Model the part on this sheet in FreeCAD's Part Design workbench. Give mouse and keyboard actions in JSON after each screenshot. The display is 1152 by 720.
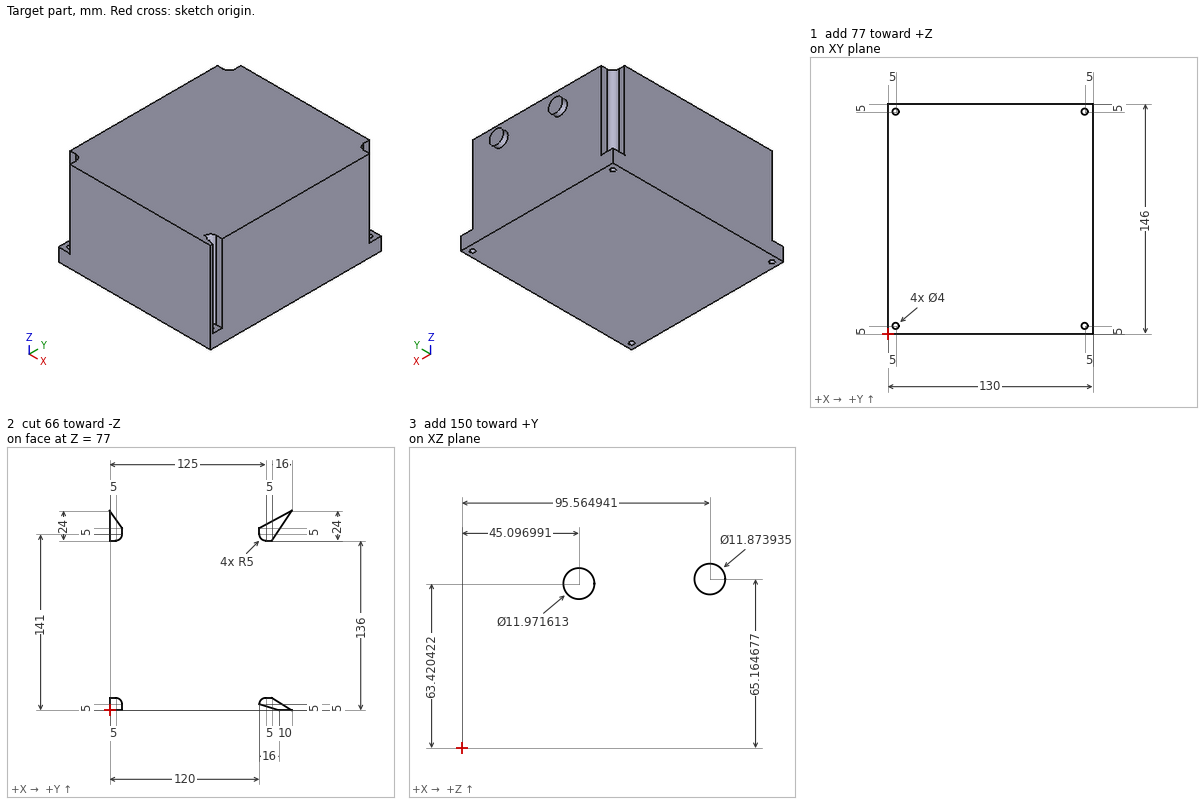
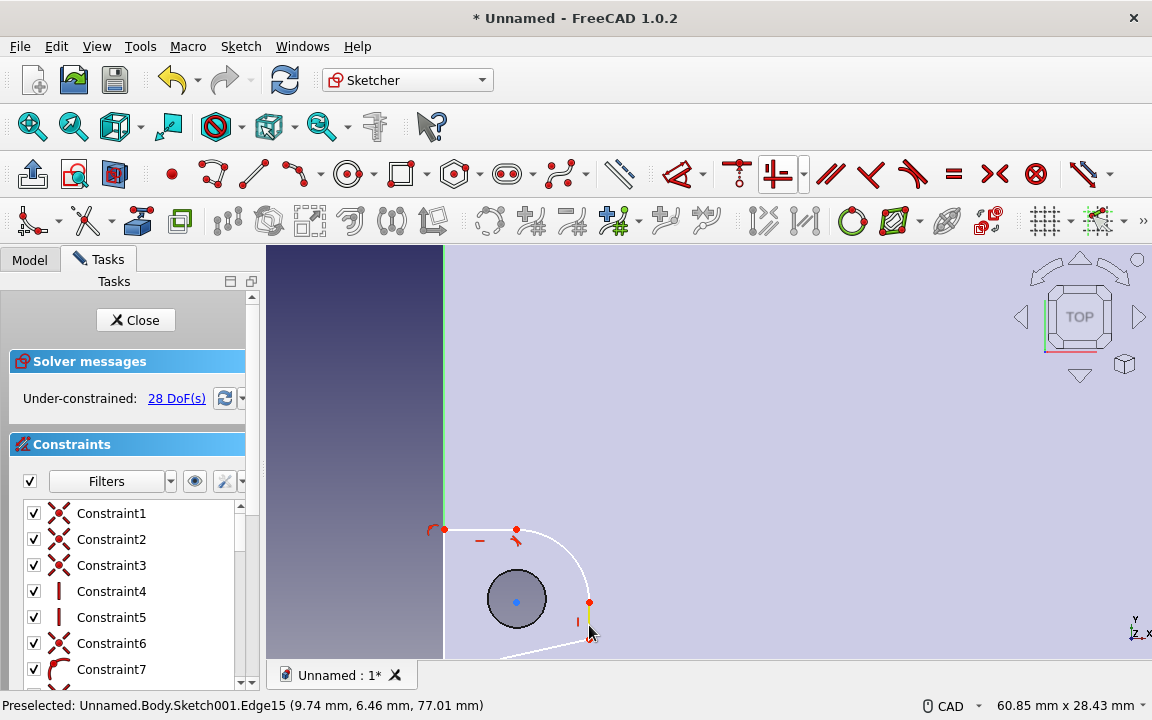
{"action": "left_click", "coordinate": [589, 625]}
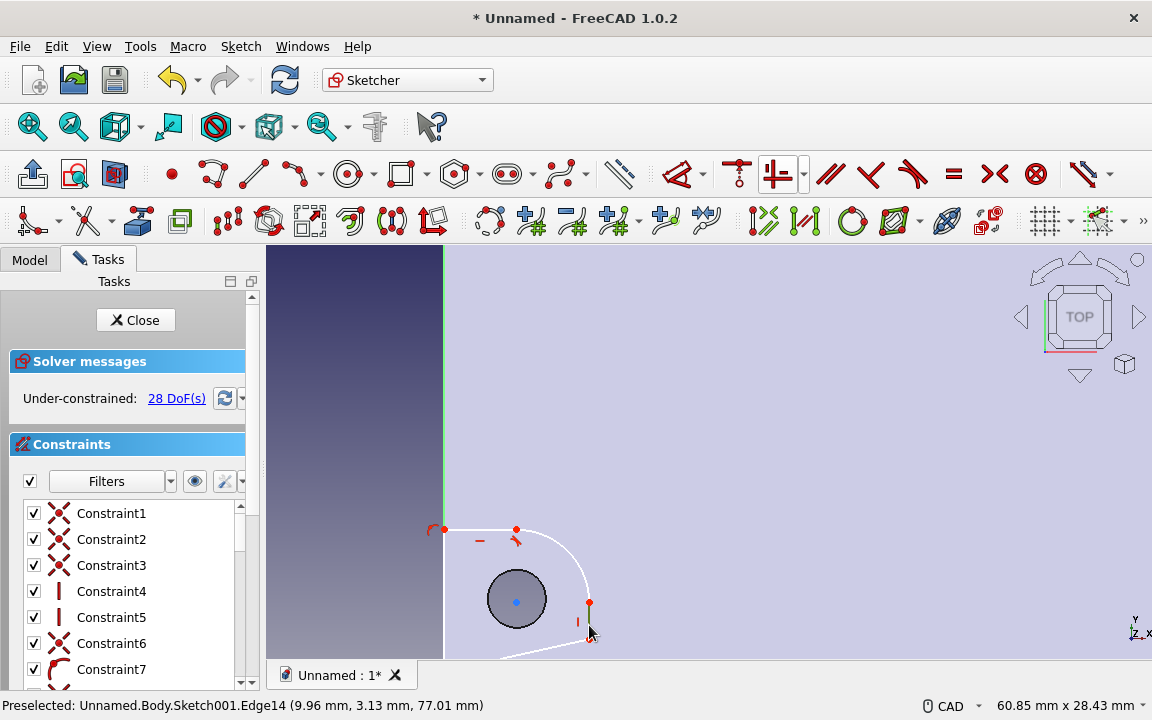
{"action": "left_click", "coordinate": [581, 570]}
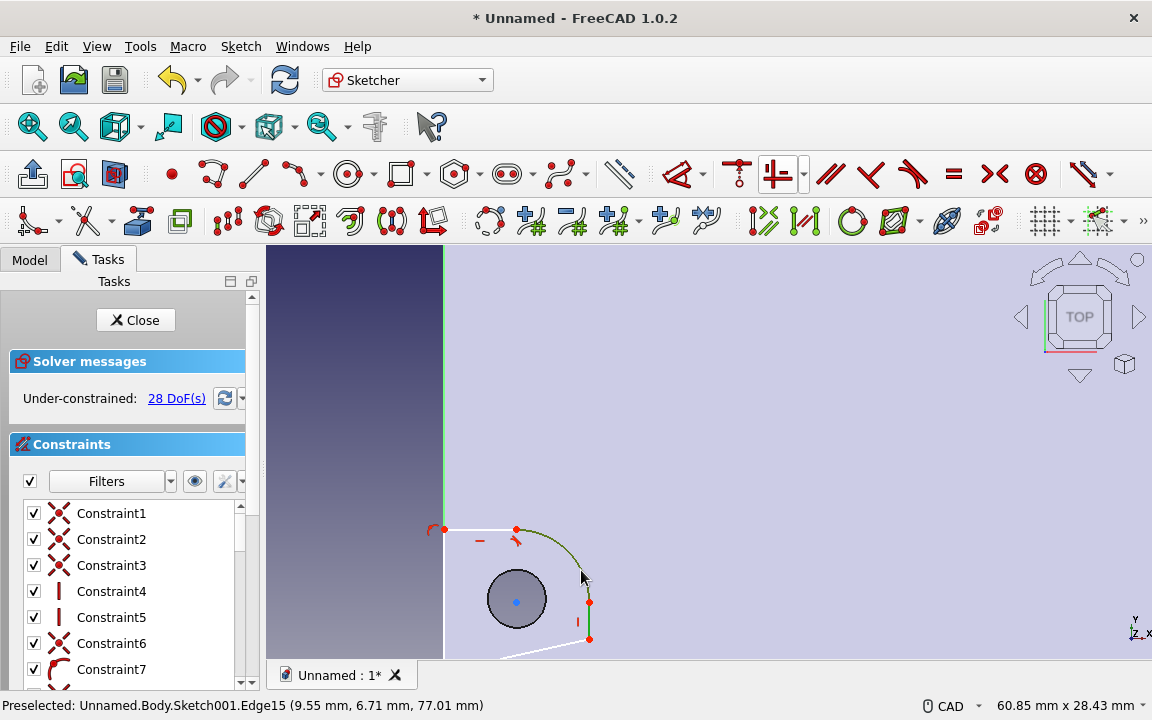
{"action": "left_click", "coordinate": [913, 174]}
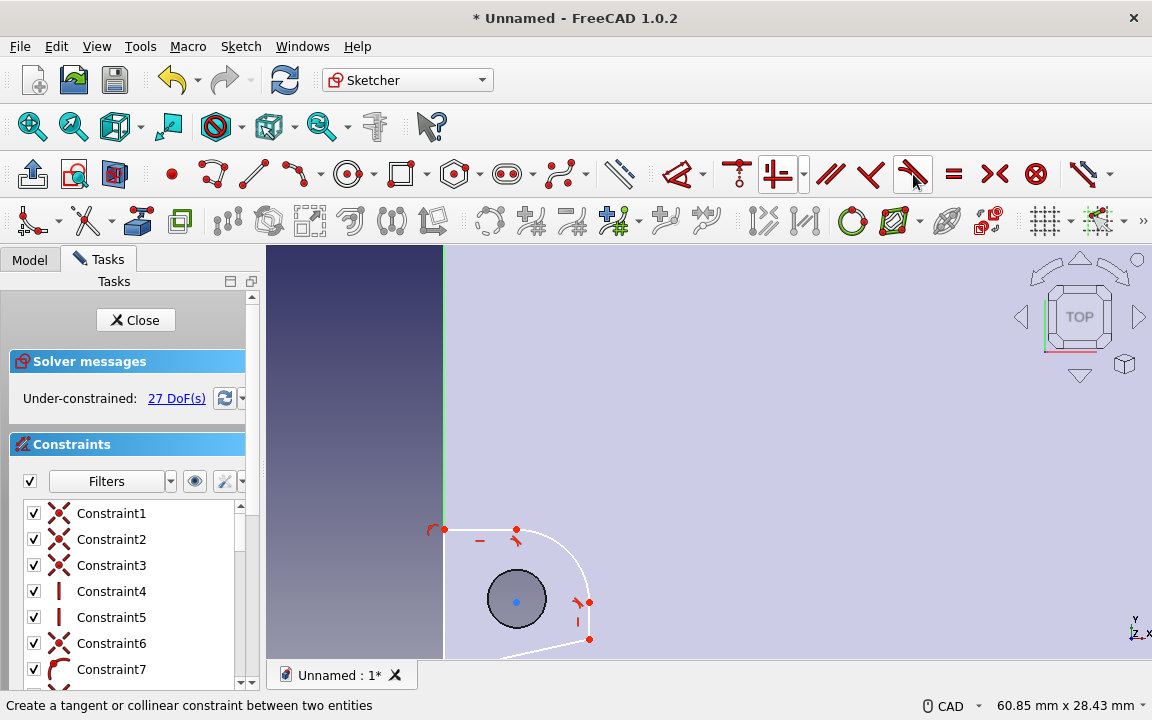
{"action": "scroll", "coordinate": [533, 570], "scroll_direction": "down", "scroll_amount": 11}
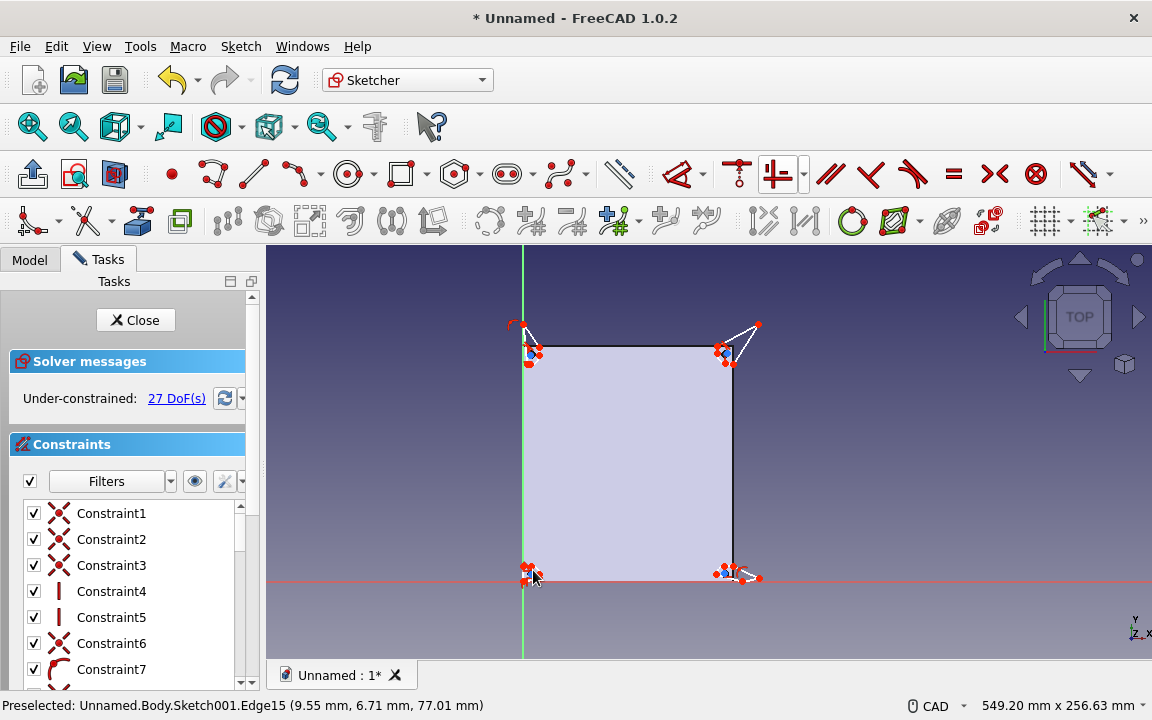
{"action": "scroll", "coordinate": [731, 566], "scroll_direction": "up", "scroll_amount": 9}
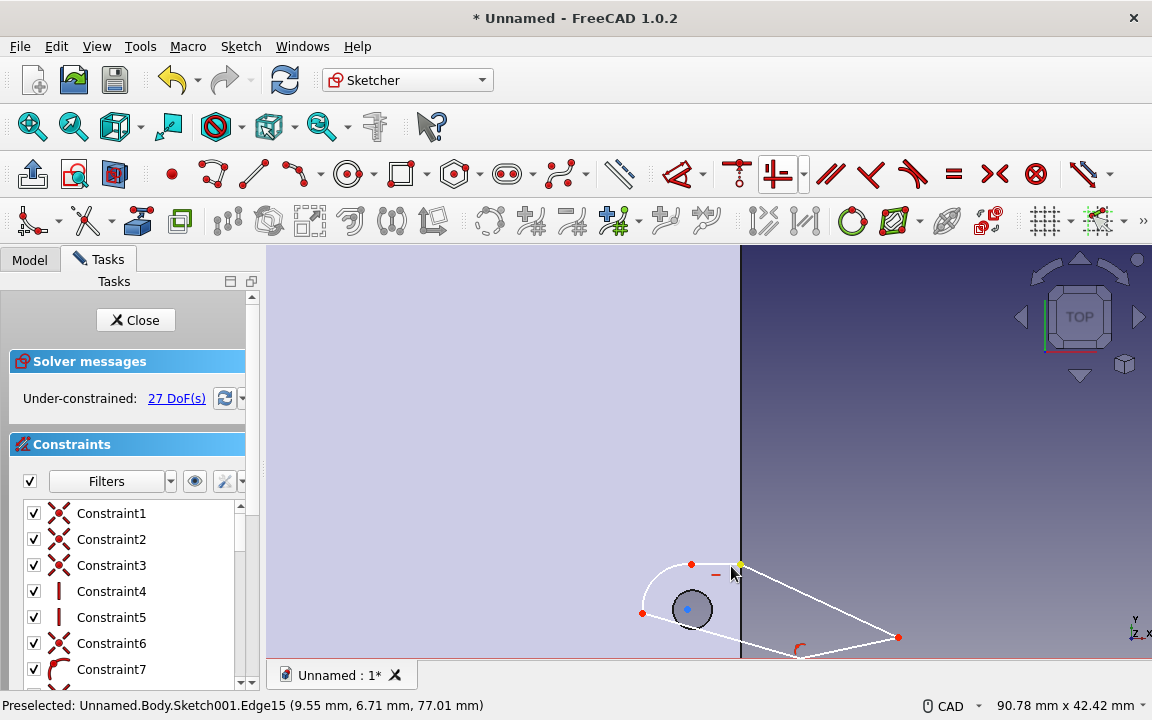
{"action": "left_click", "coordinate": [726, 564]}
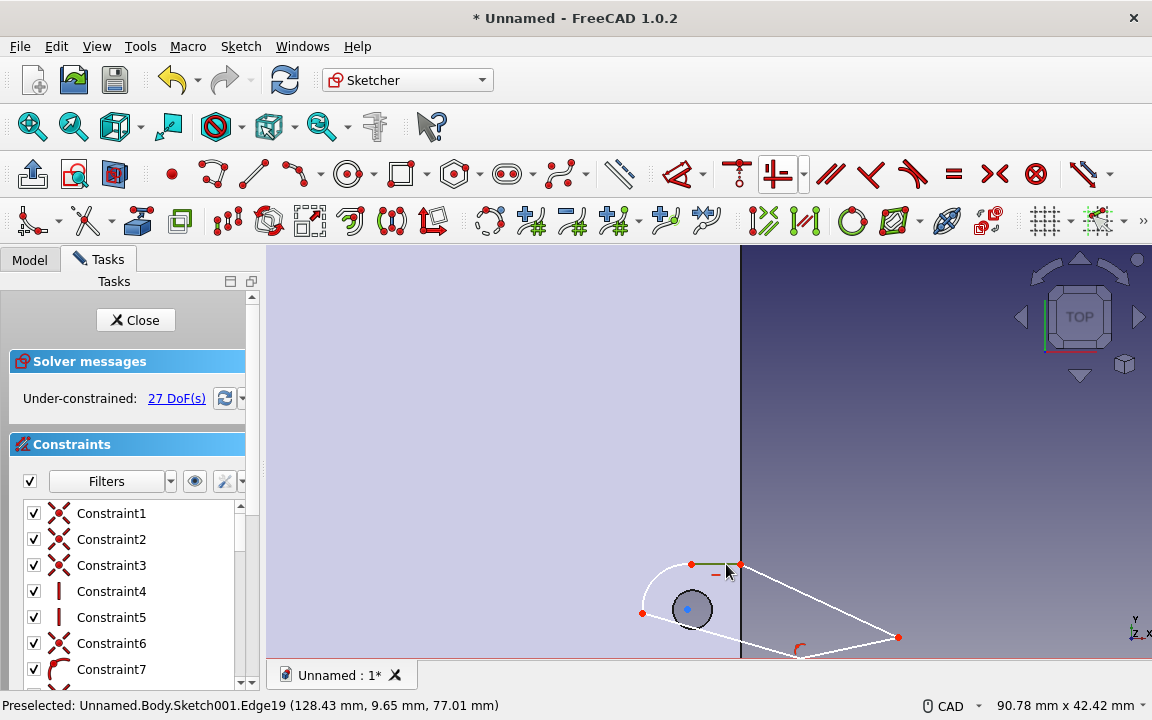
{"action": "left_click", "coordinate": [669, 568]}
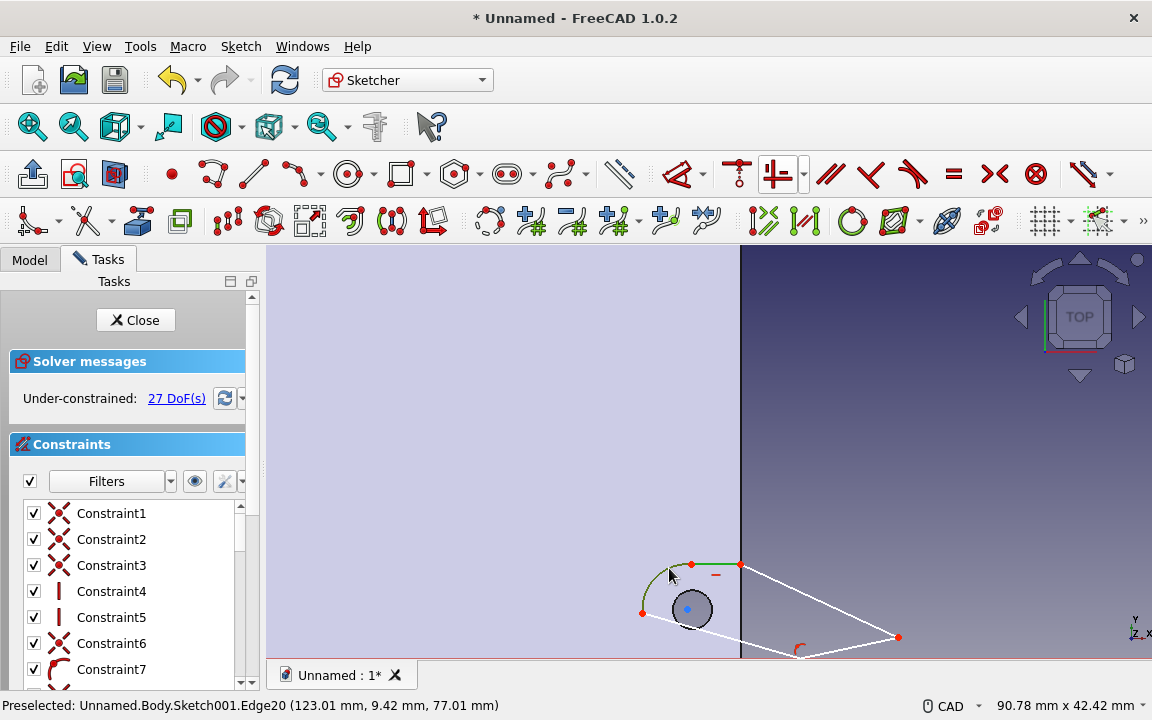
{"action": "left_click", "coordinate": [913, 174]}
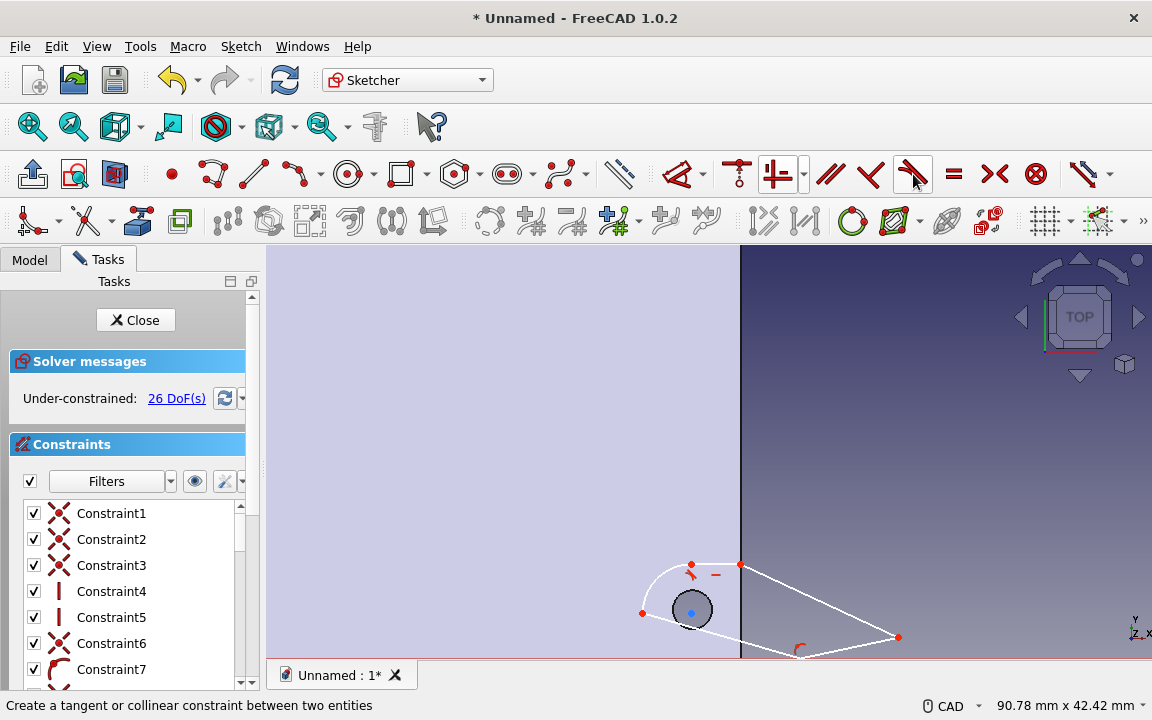
{"action": "scroll", "coordinate": [731, 566], "scroll_direction": "down", "scroll_amount": 9}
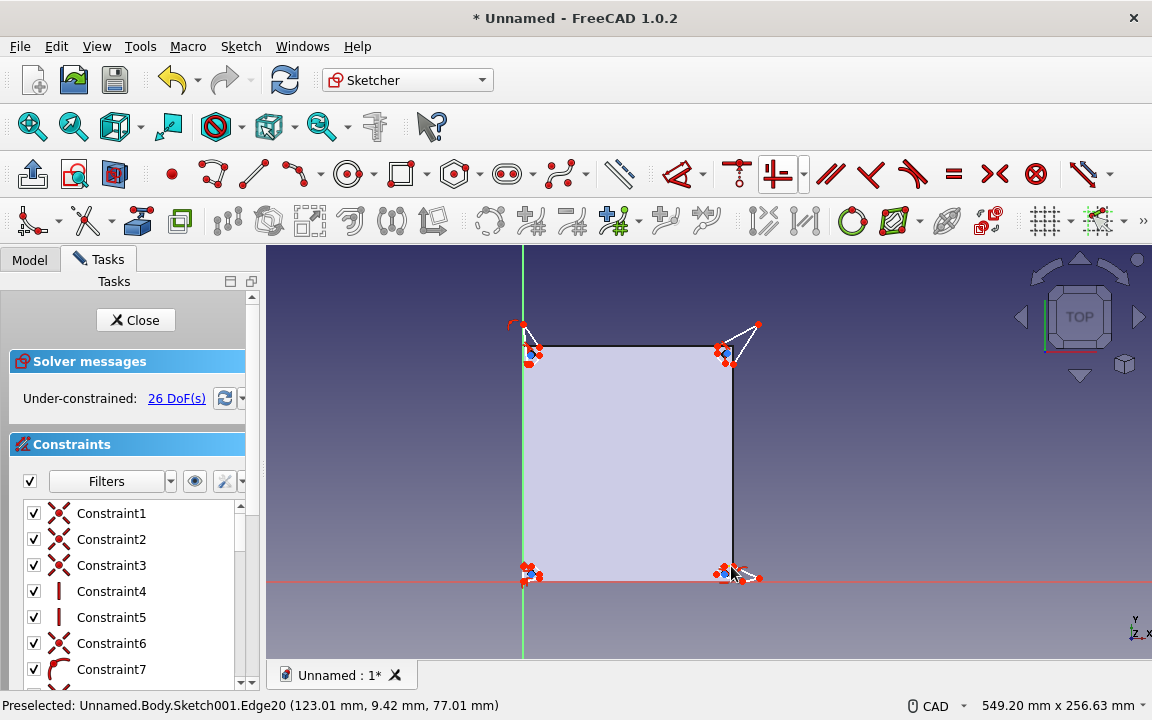
{"action": "scroll", "coordinate": [728, 364], "scroll_direction": "up", "scroll_amount": 9}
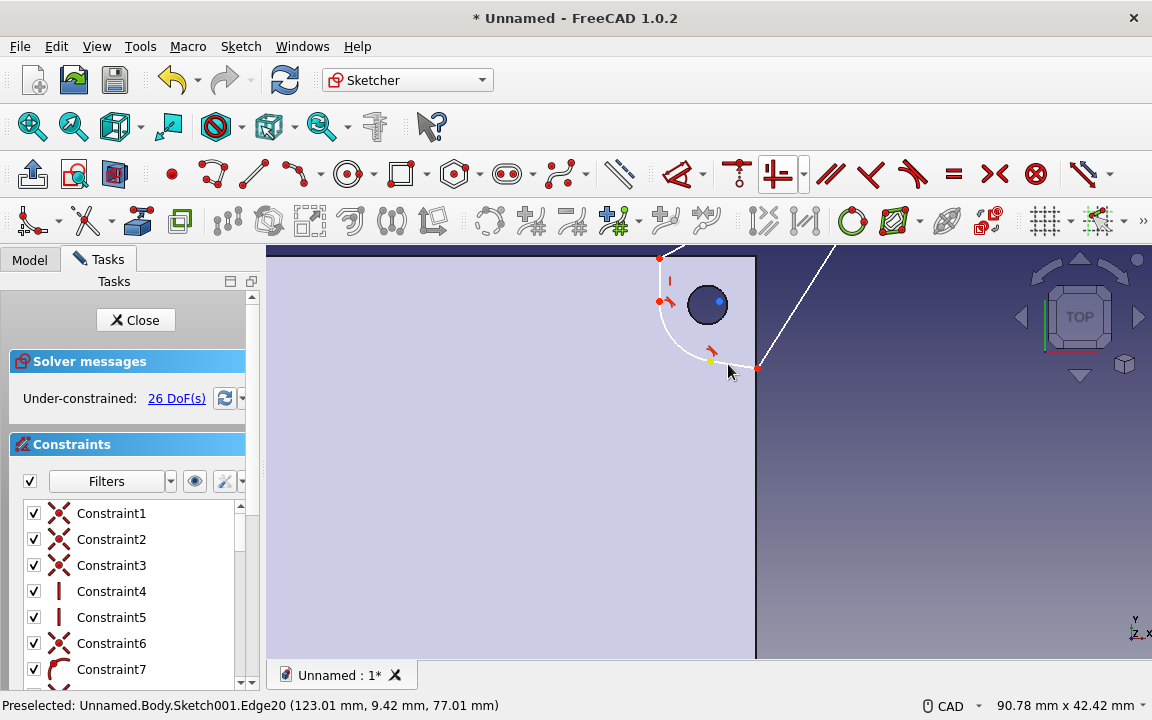
{"action": "left_click", "coordinate": [725, 363]}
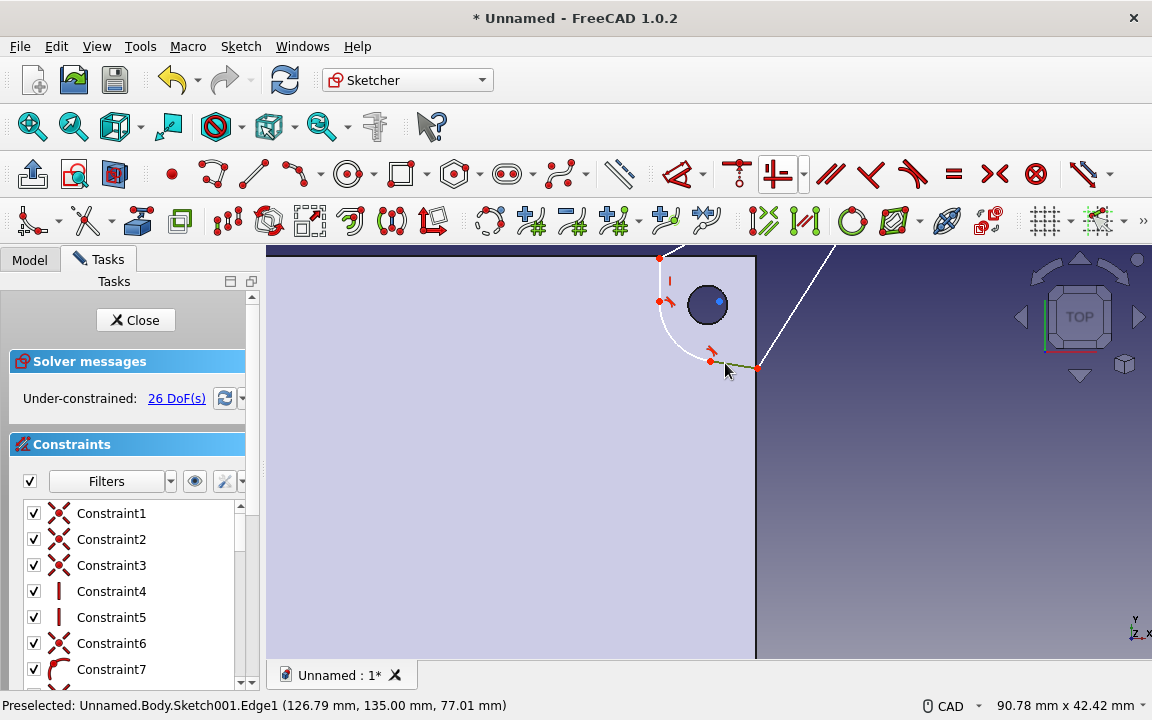
{"action": "key", "text": "h"}